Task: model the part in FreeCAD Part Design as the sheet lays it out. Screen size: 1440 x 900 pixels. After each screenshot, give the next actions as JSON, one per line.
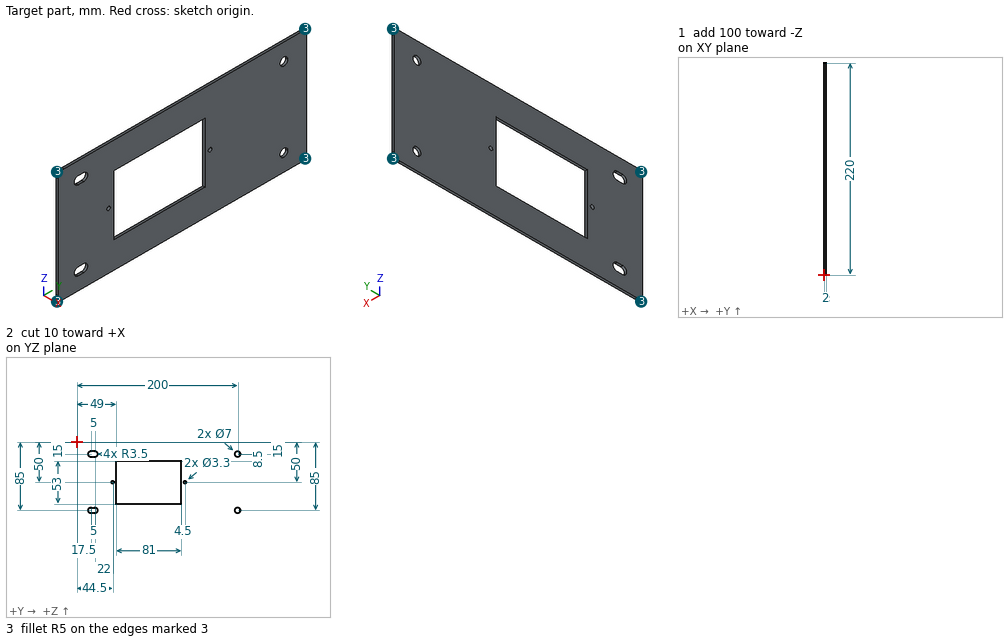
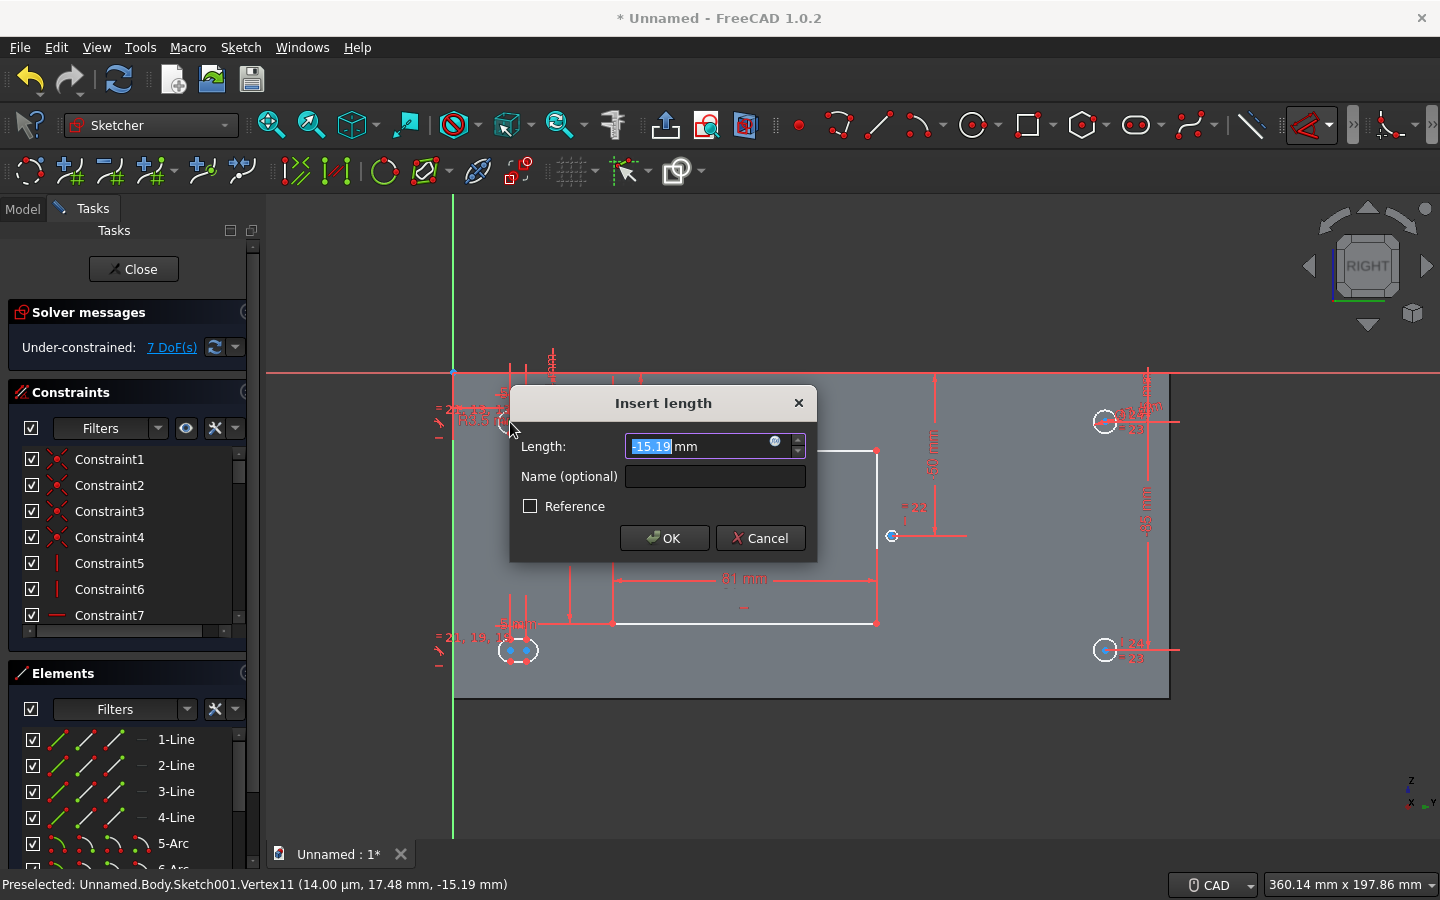
{"action": "type", "text": "-15"}
{"action": "key", "text": "Return"}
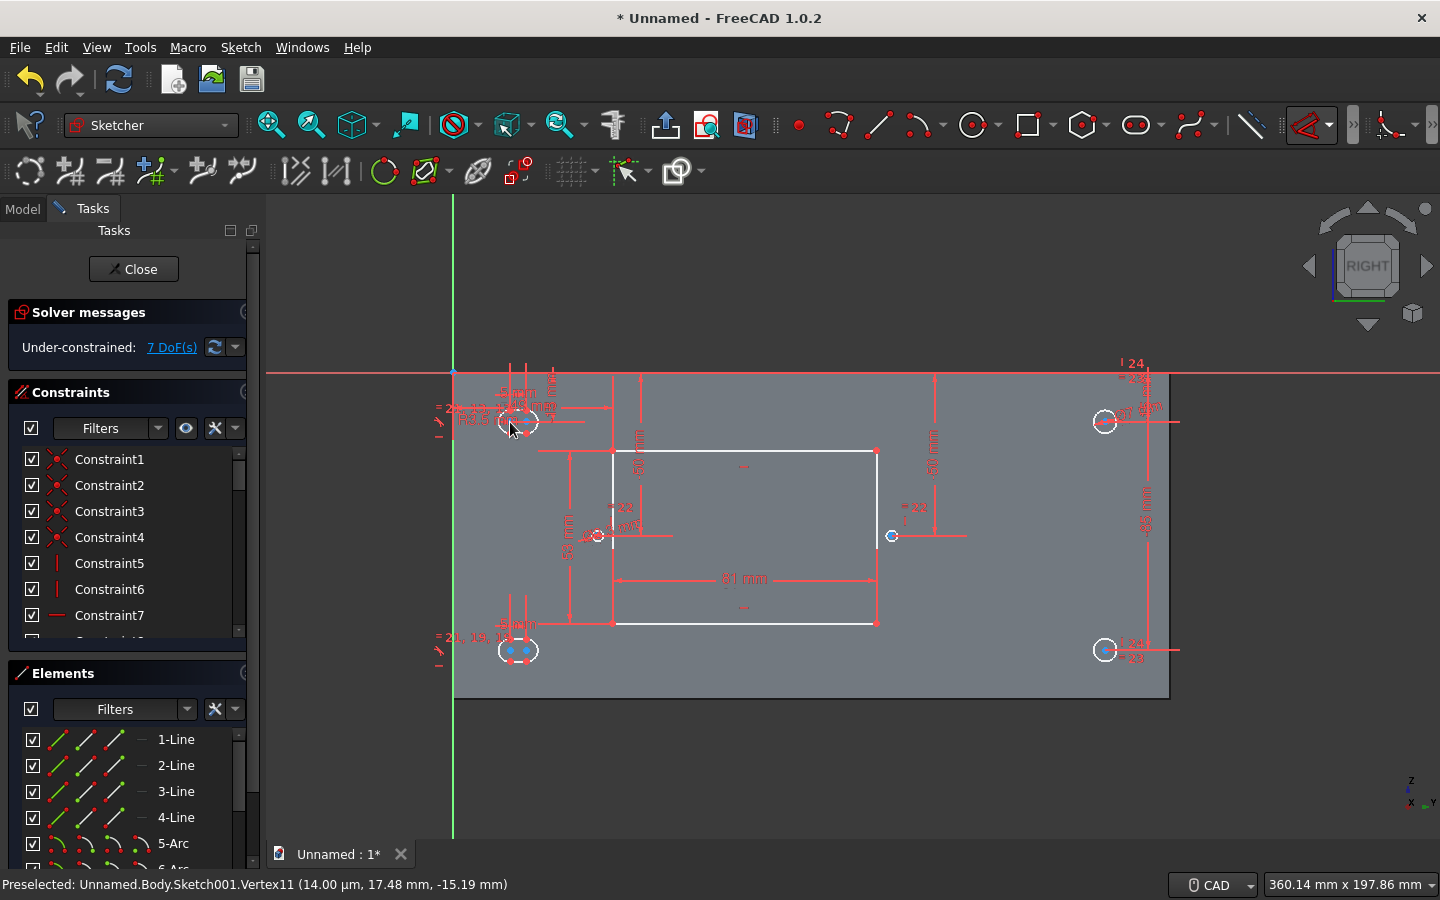
{"action": "left_click", "coordinate": [512, 653]}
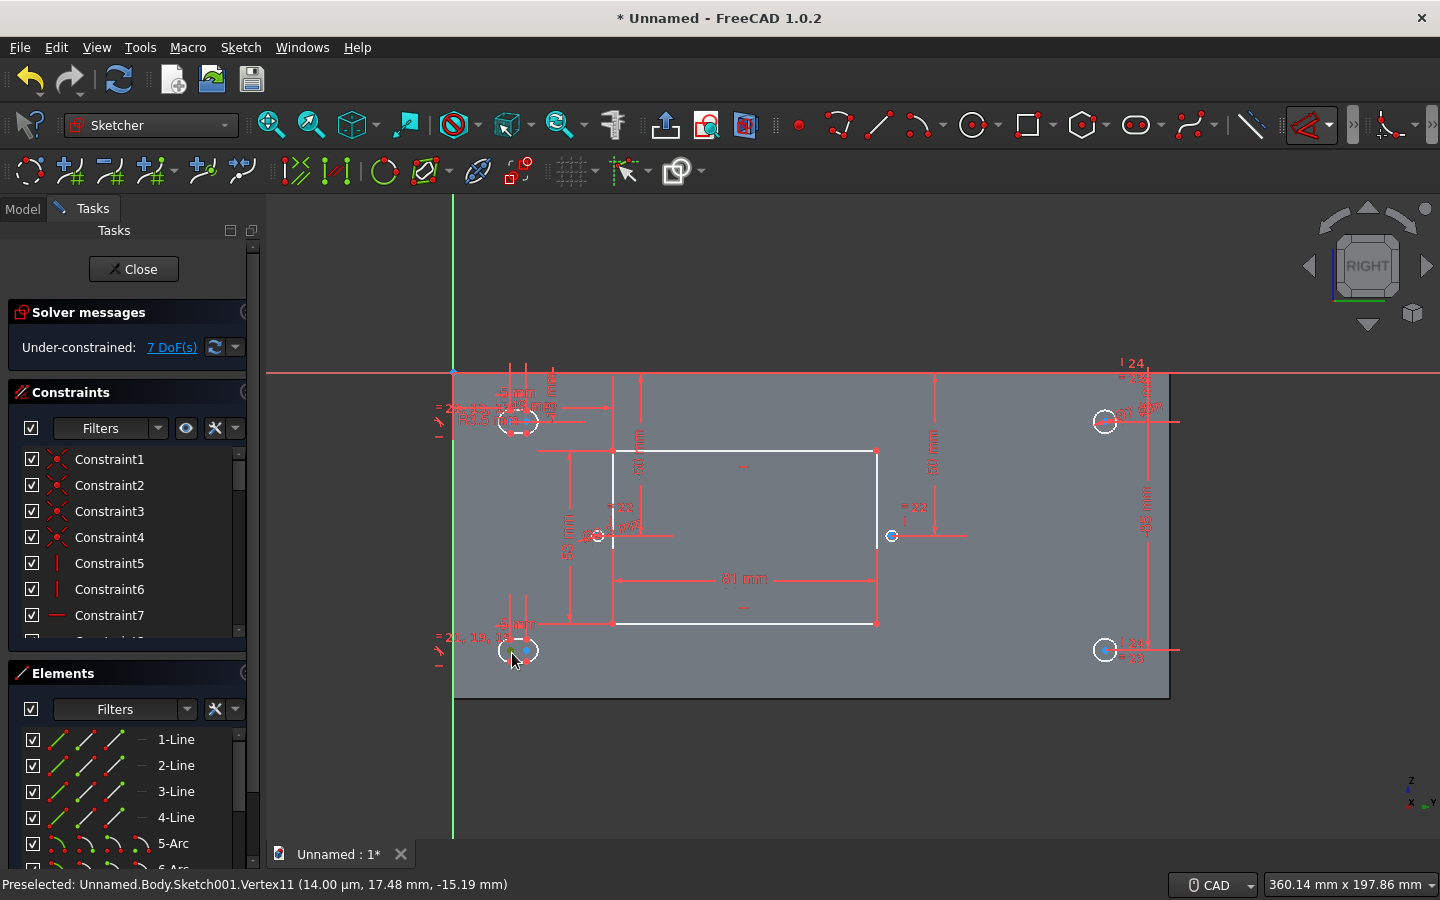
{"action": "left_click", "coordinate": [1332, 126]}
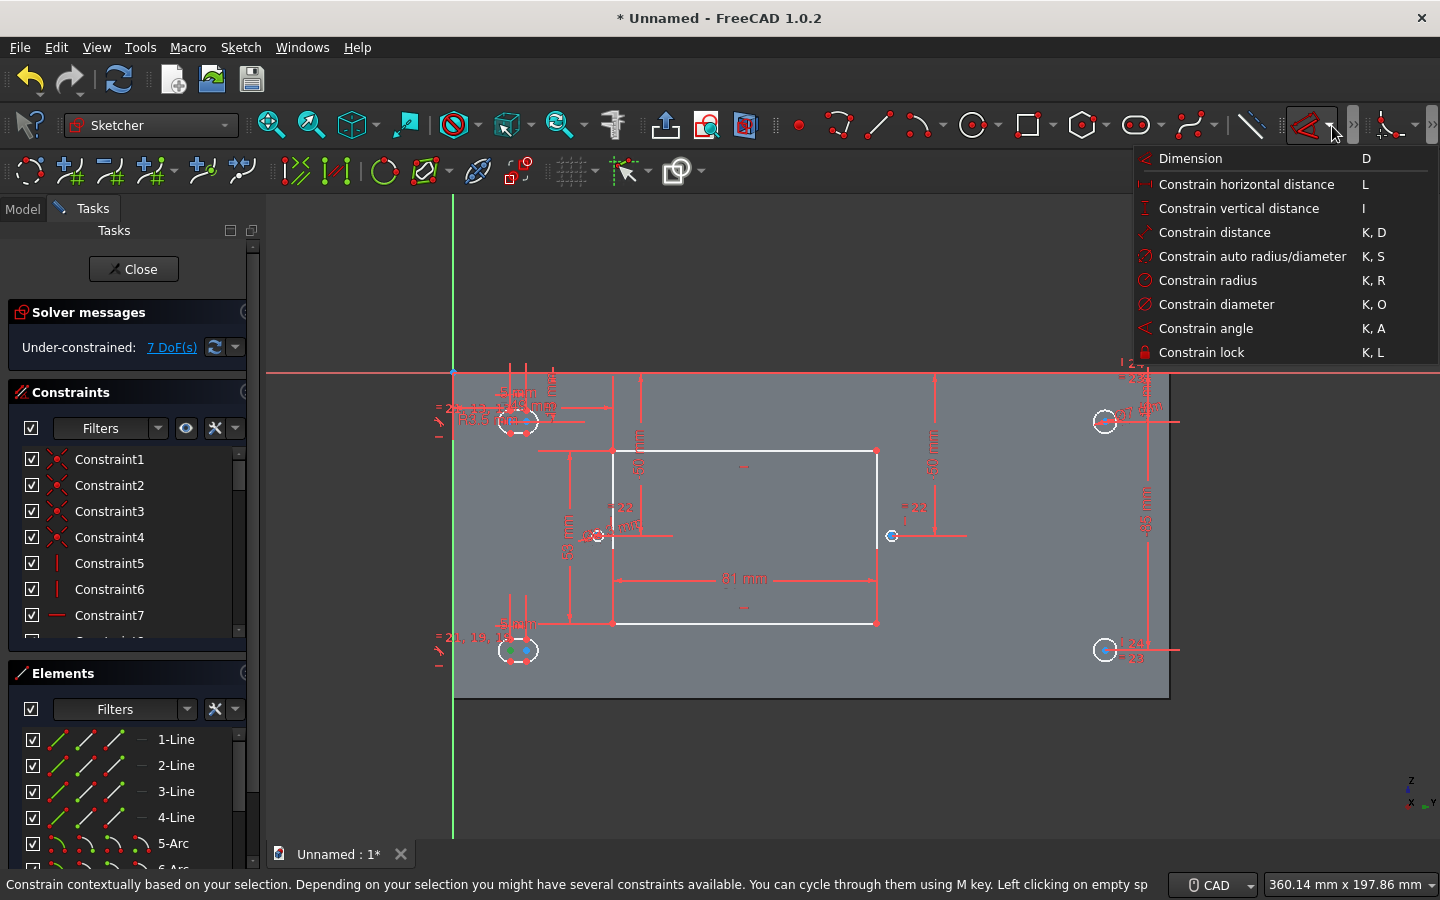
{"action": "left_click", "coordinate": [1286, 208]}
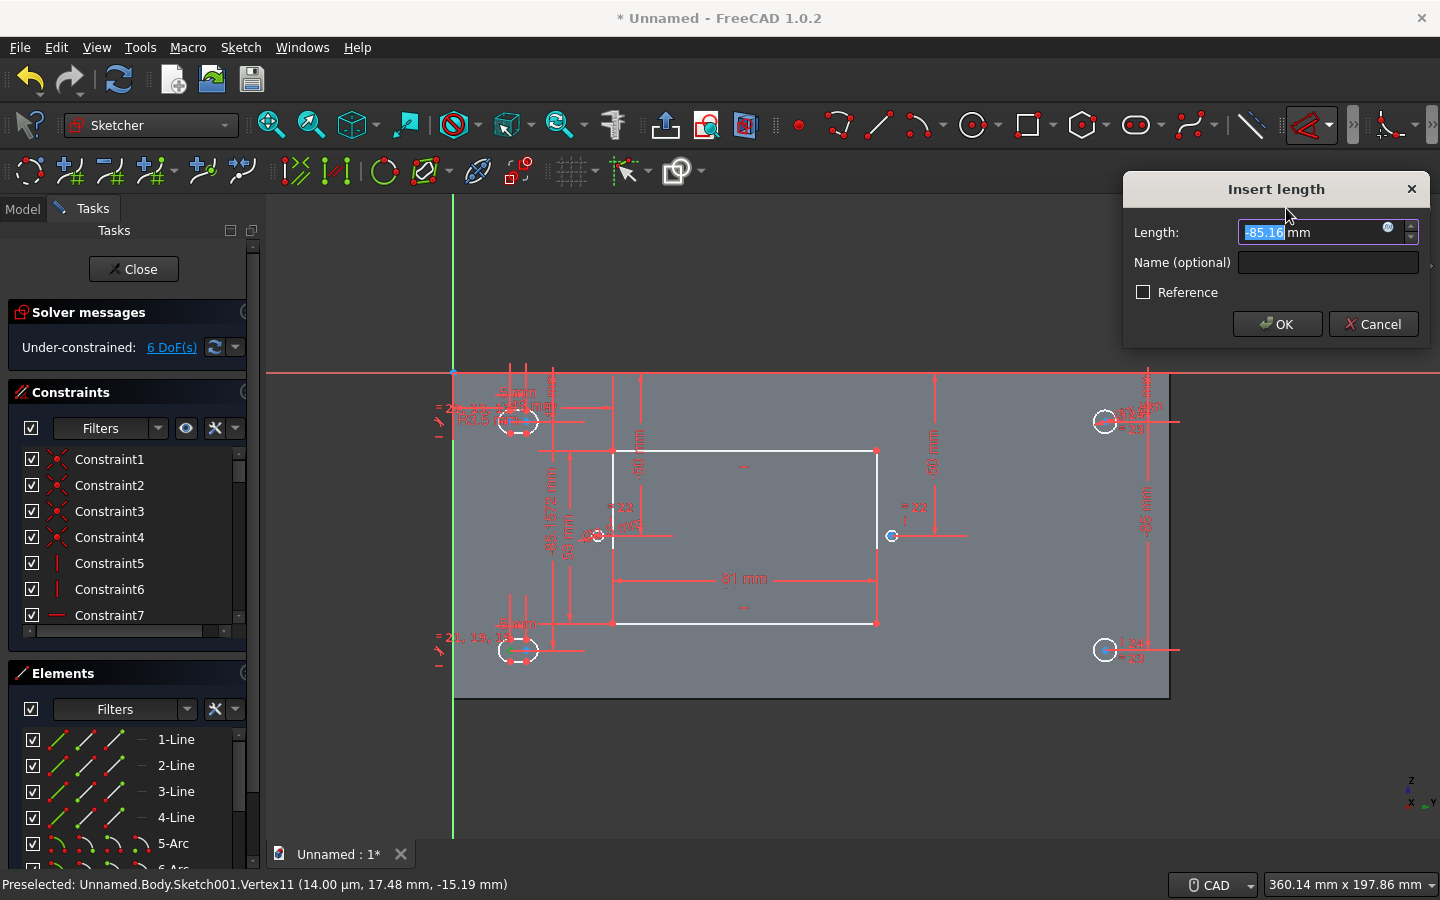
{"action": "type", "text": "-85"}
{"action": "key", "text": "Return"}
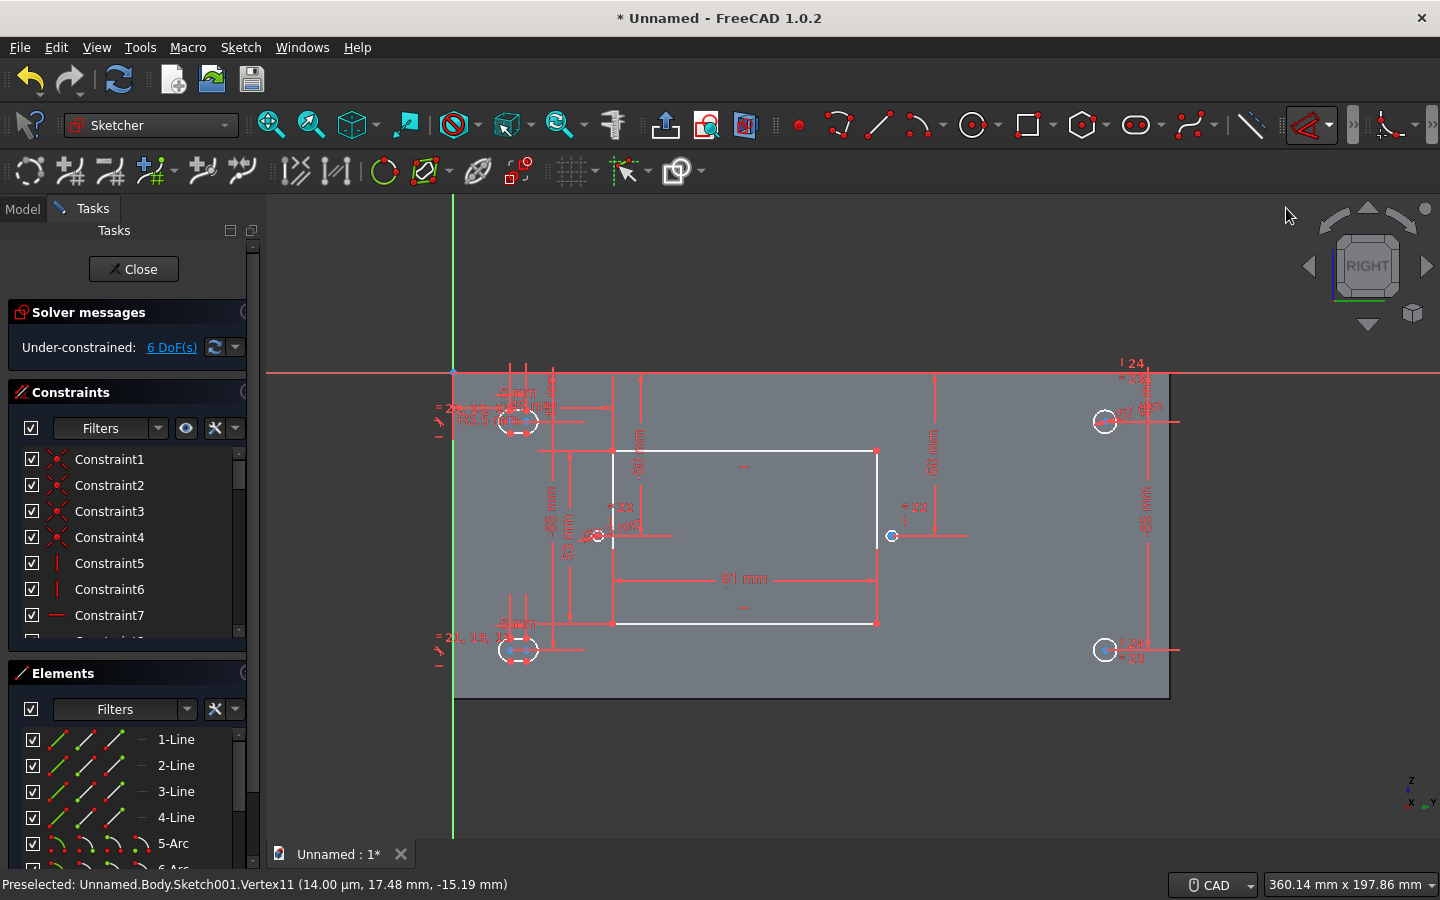
{"action": "left_click", "coordinate": [1105, 422]}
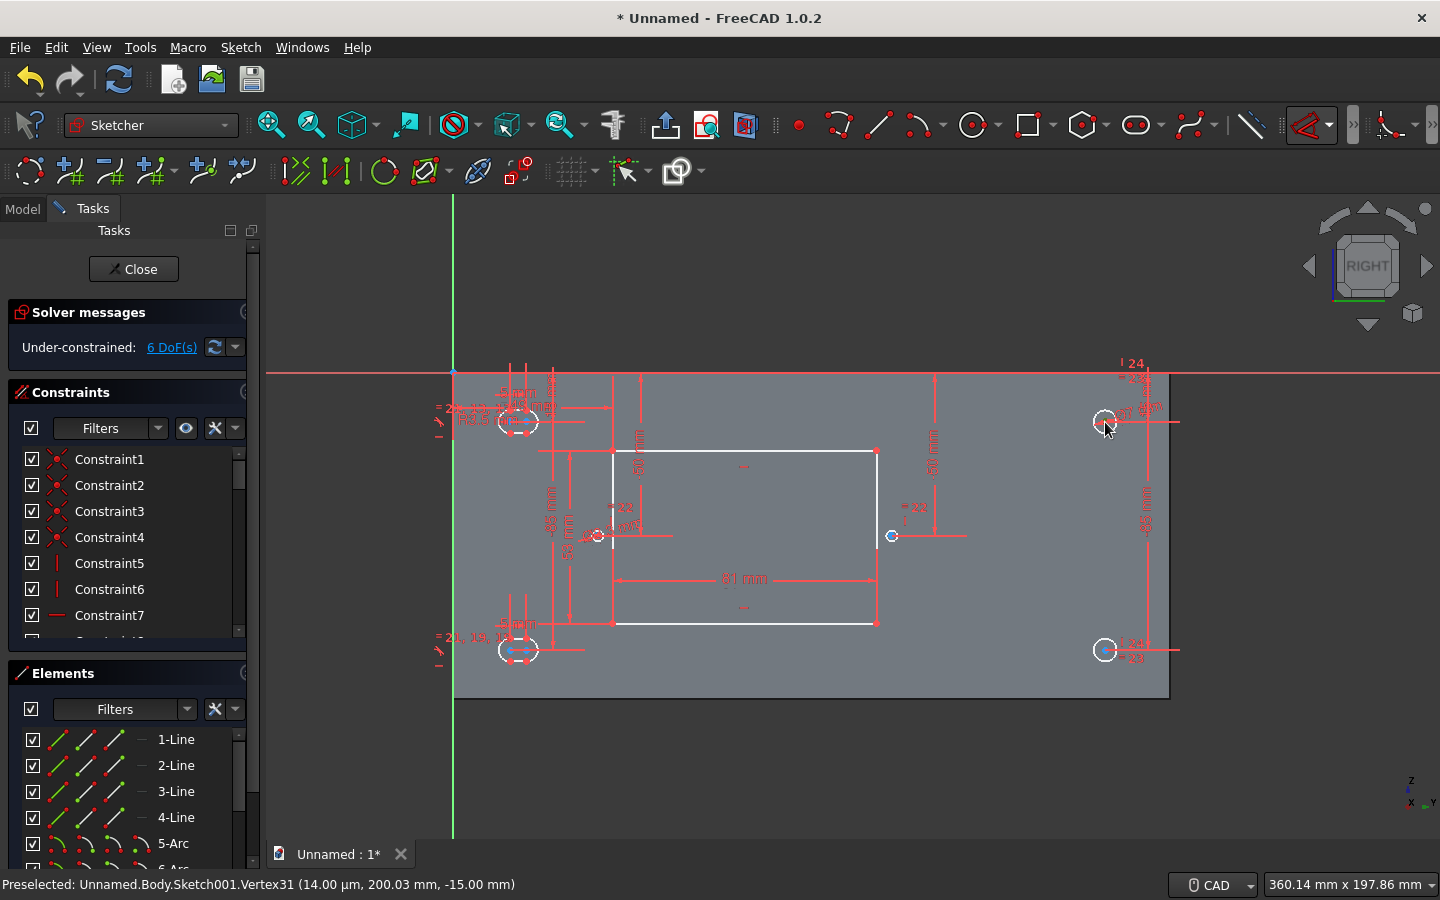
{"action": "left_click", "coordinate": [1332, 126]}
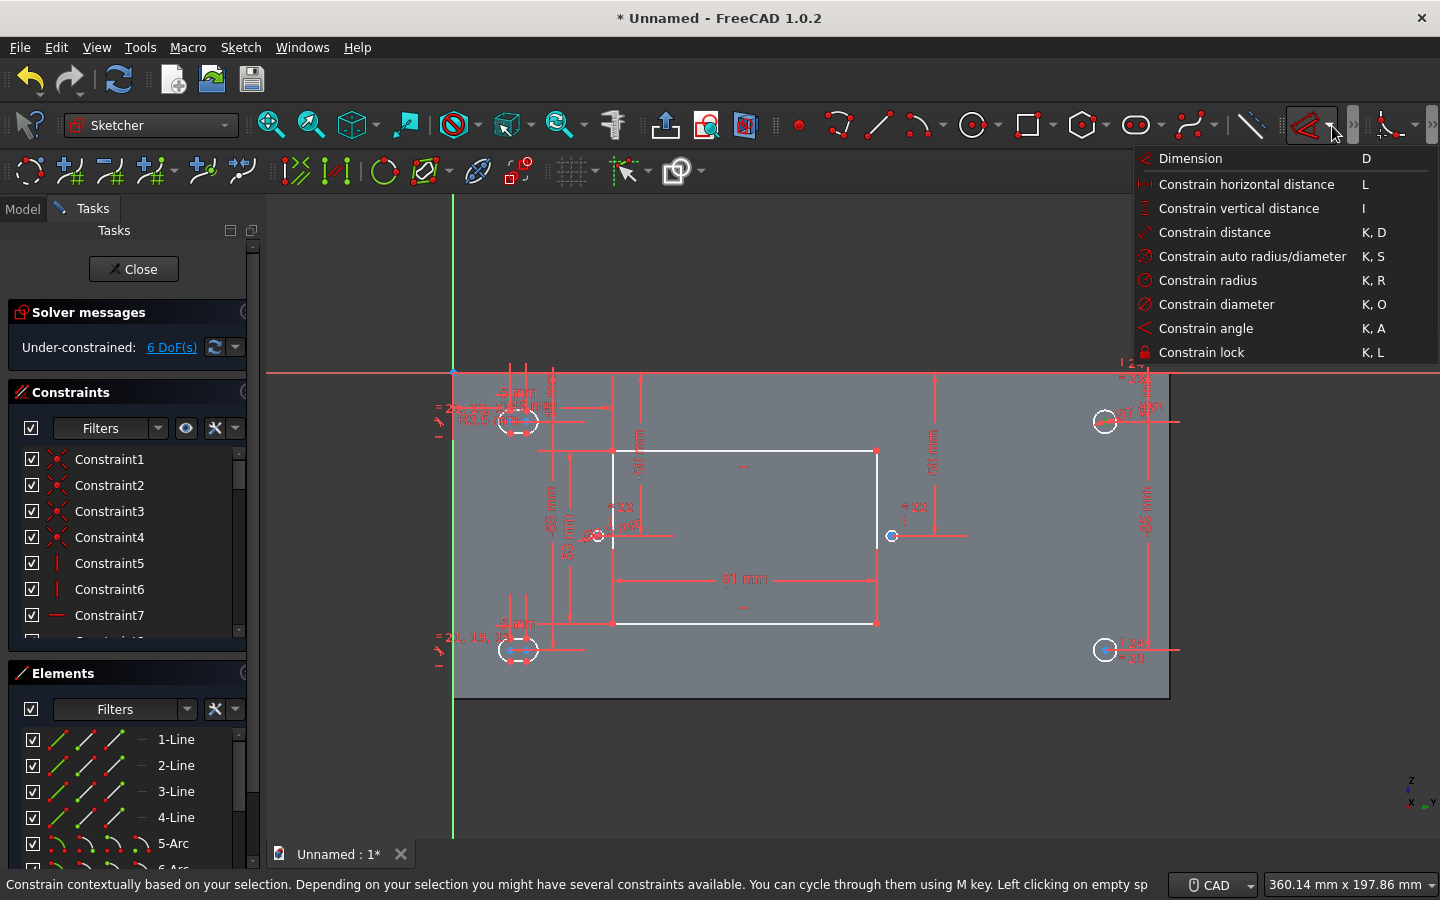
{"action": "left_click", "coordinate": [1286, 184]}